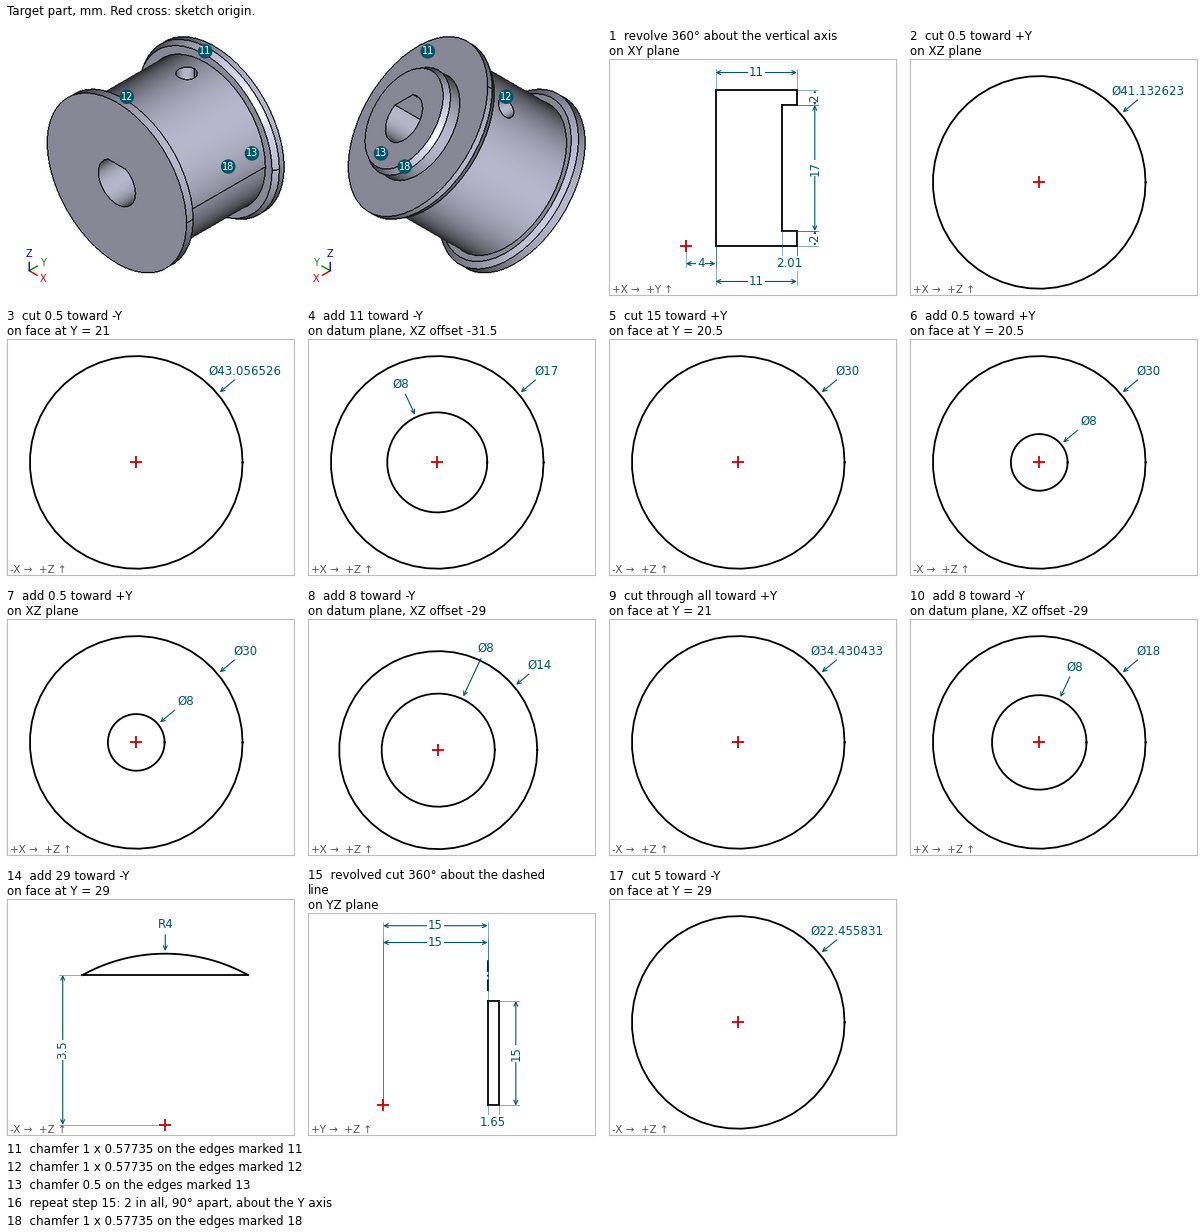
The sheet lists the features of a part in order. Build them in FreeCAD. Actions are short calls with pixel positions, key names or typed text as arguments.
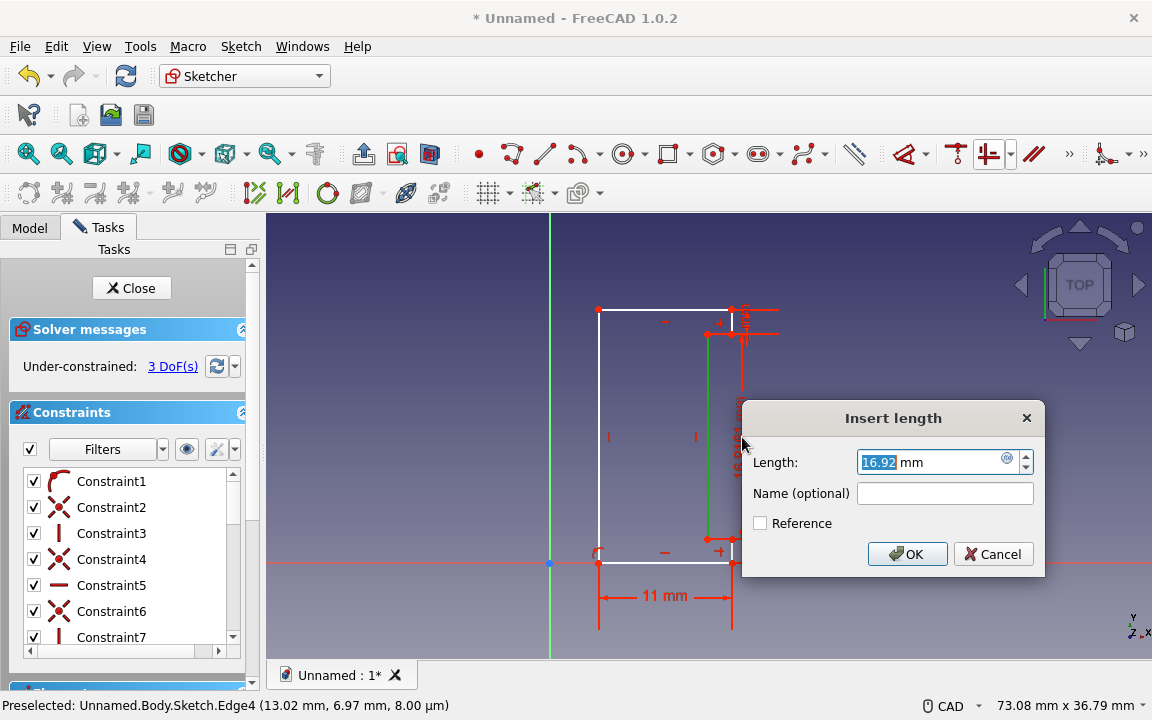
text(17)
key(Return)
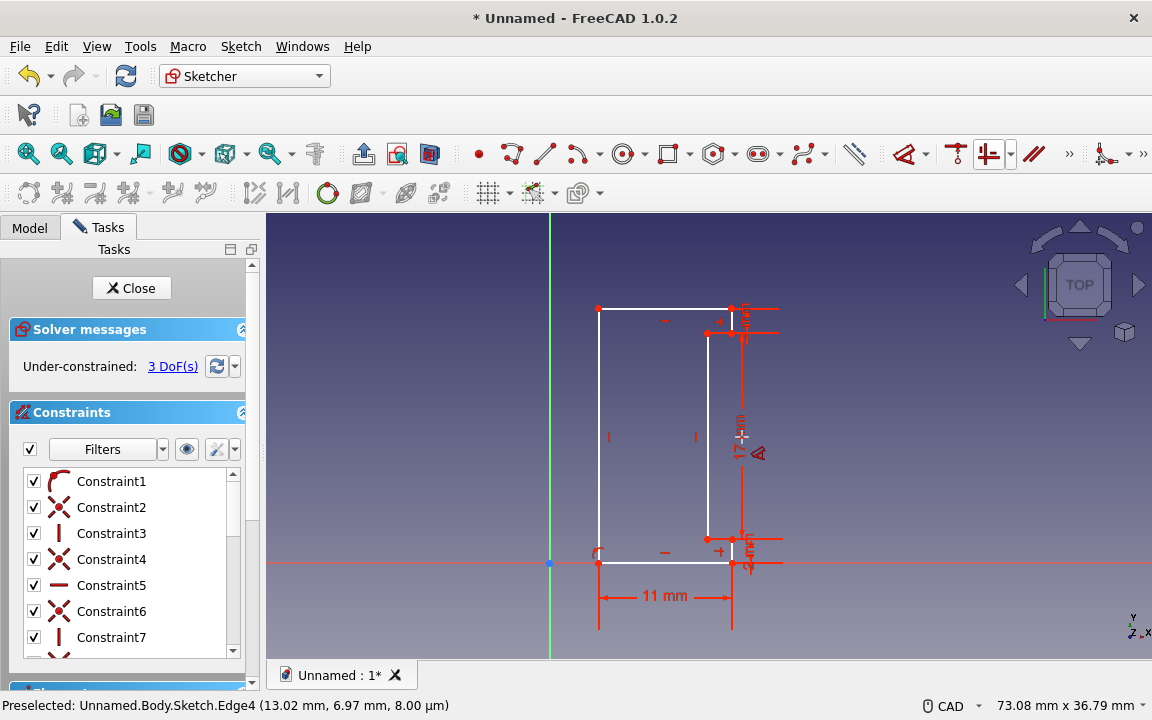
click(692, 309)
click(665, 275)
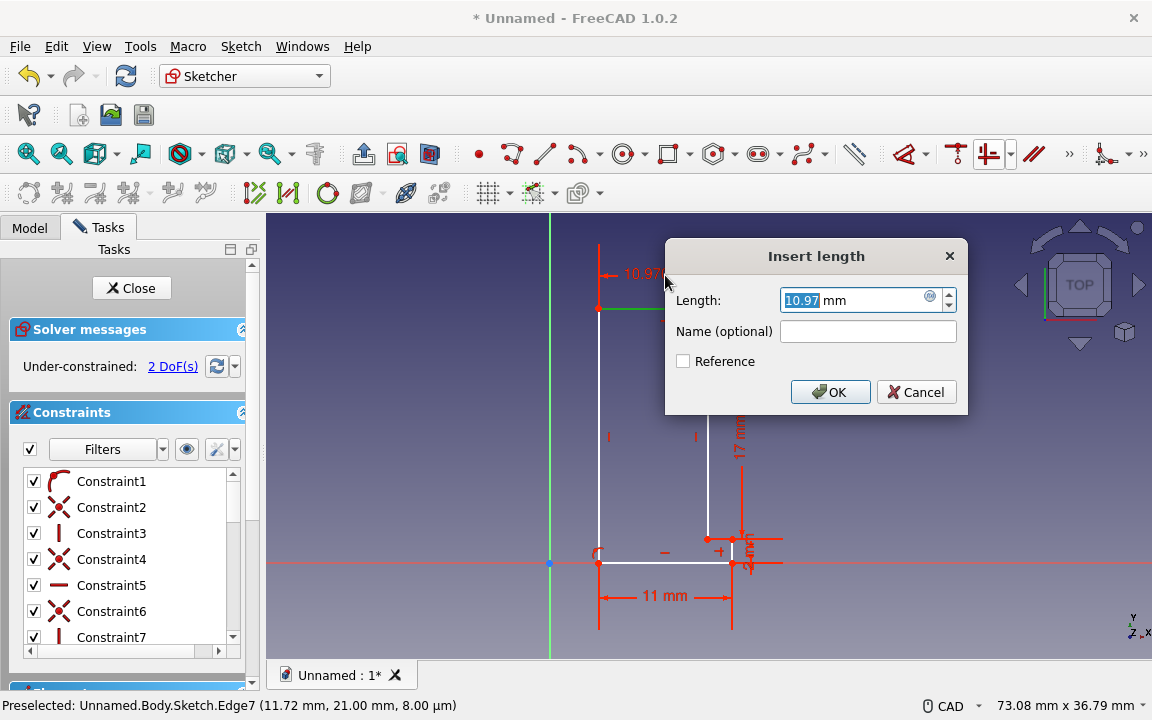
text(11)
key(Return)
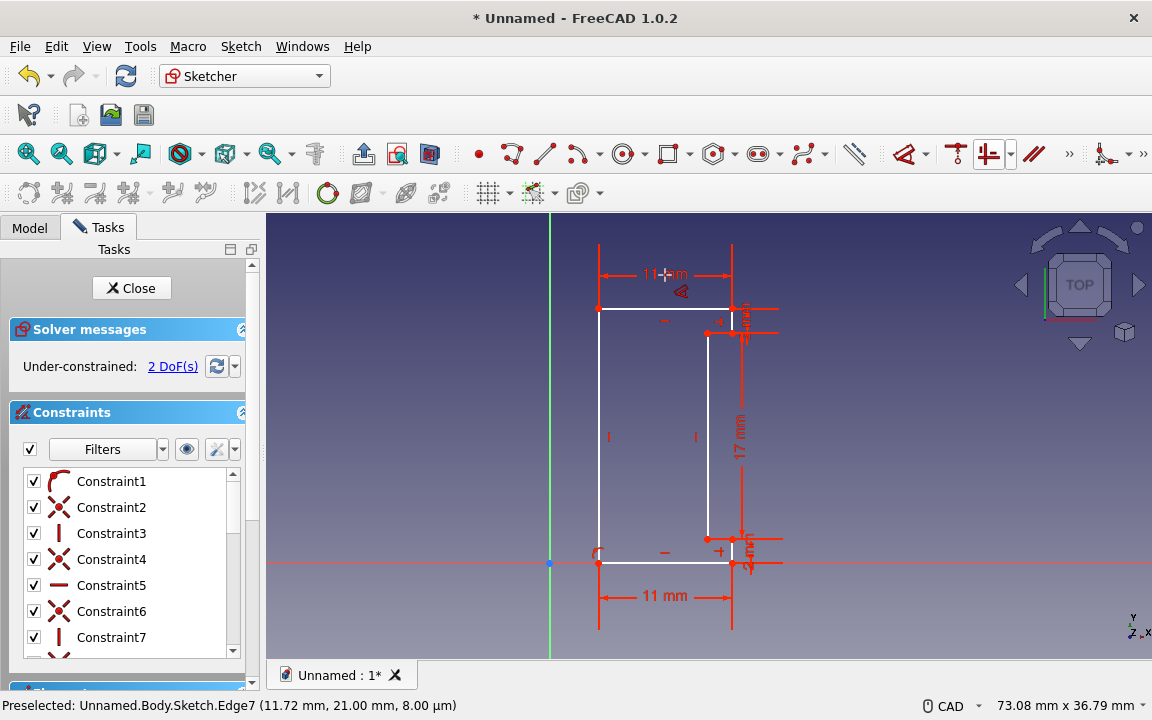
click(599, 563)
click(574, 597)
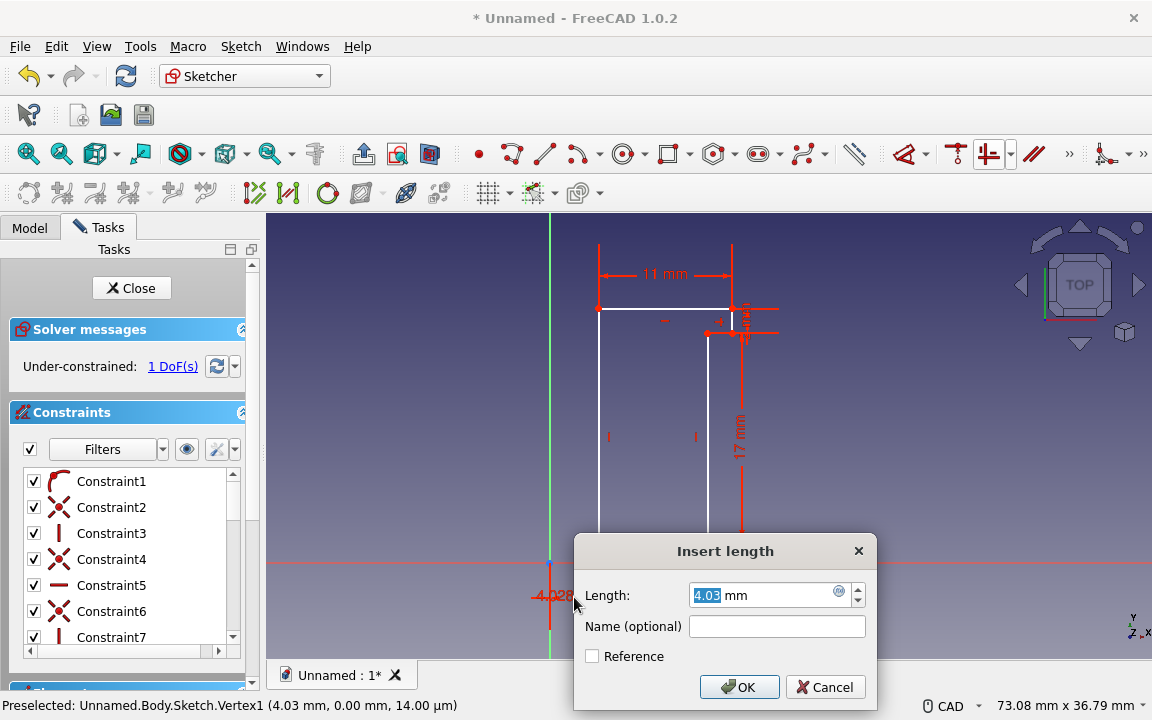
text(4)
key(Return)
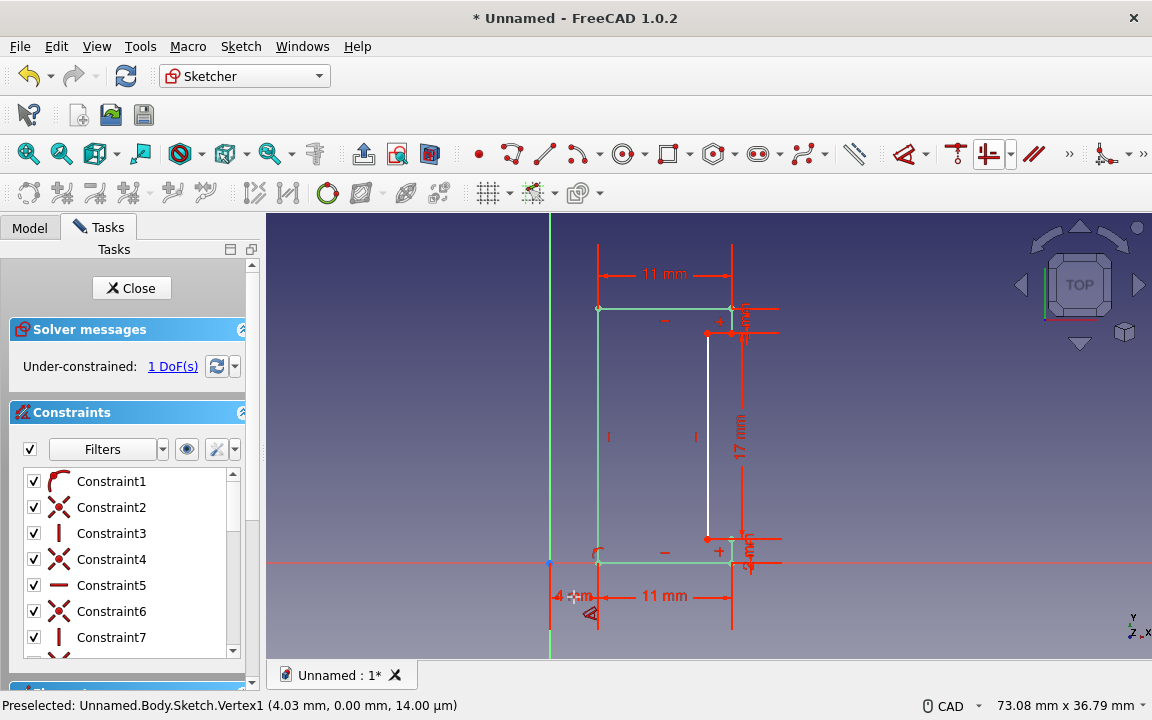
scroll(722, 539, up, 3)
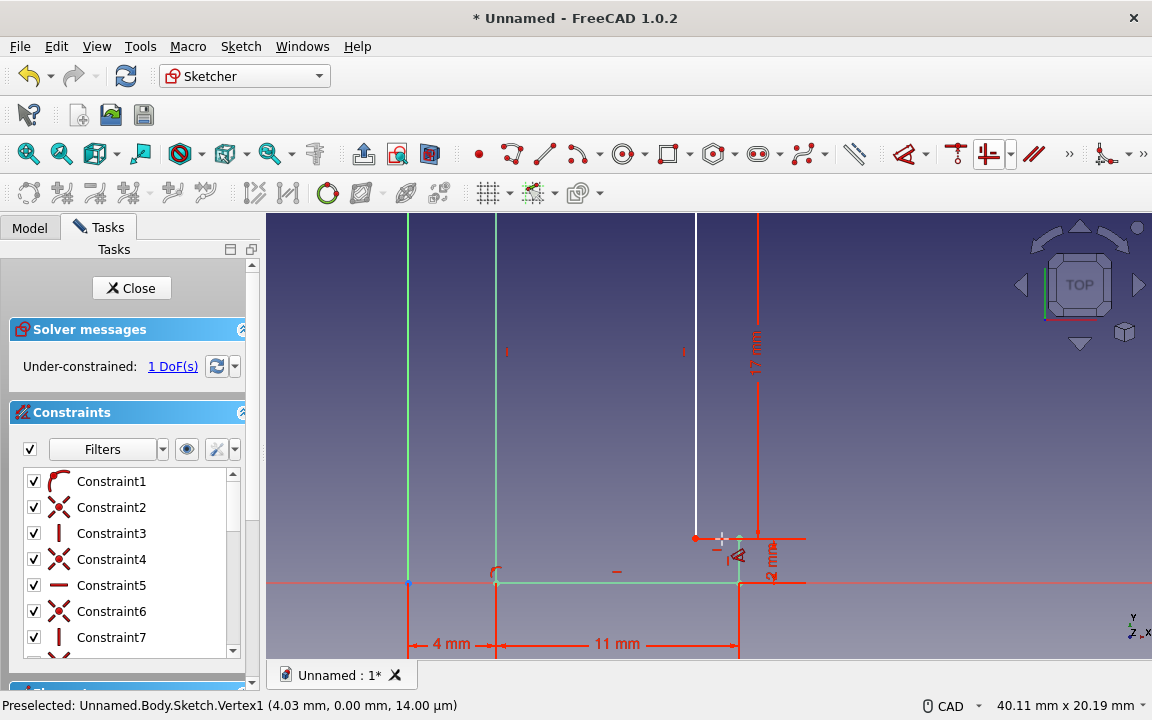
click(722, 539)
click(718, 505)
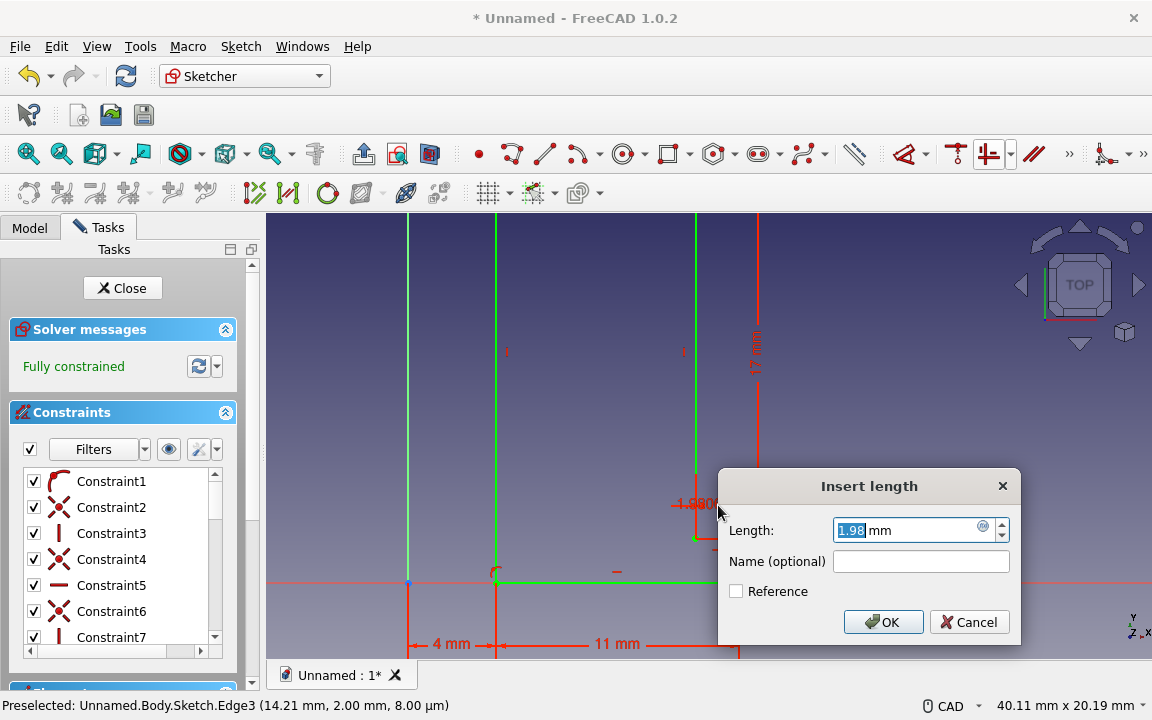
text(2.01)
key(Return)
key(Escape)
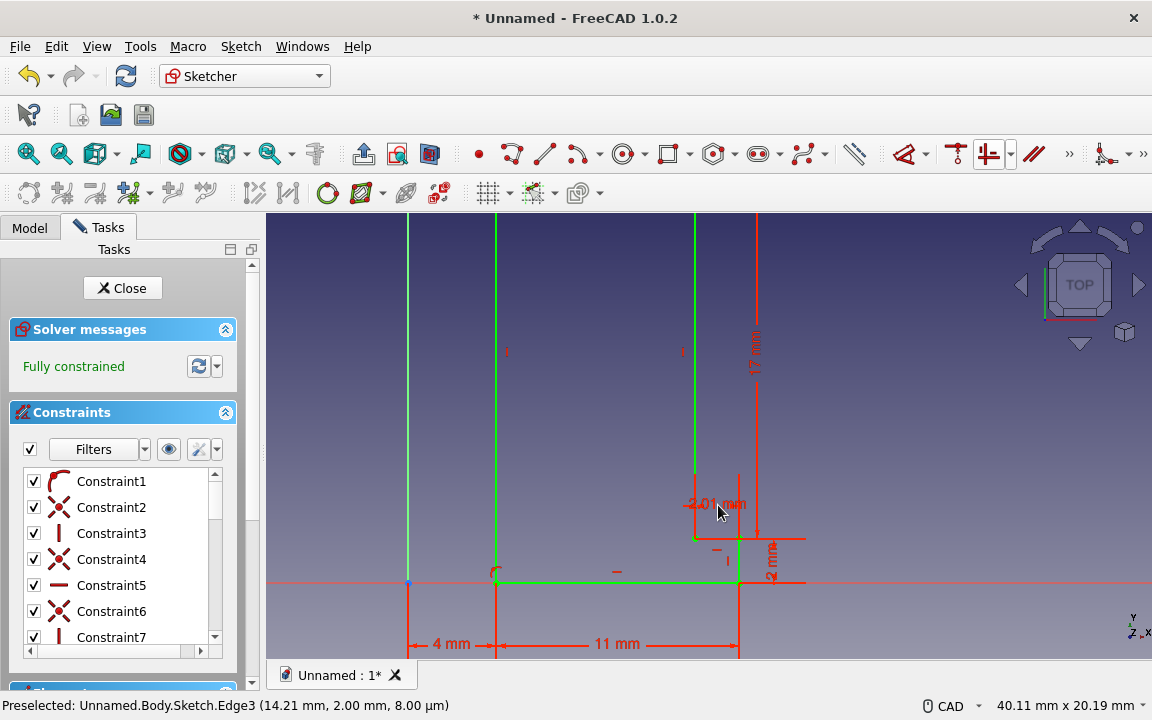
click(123, 288)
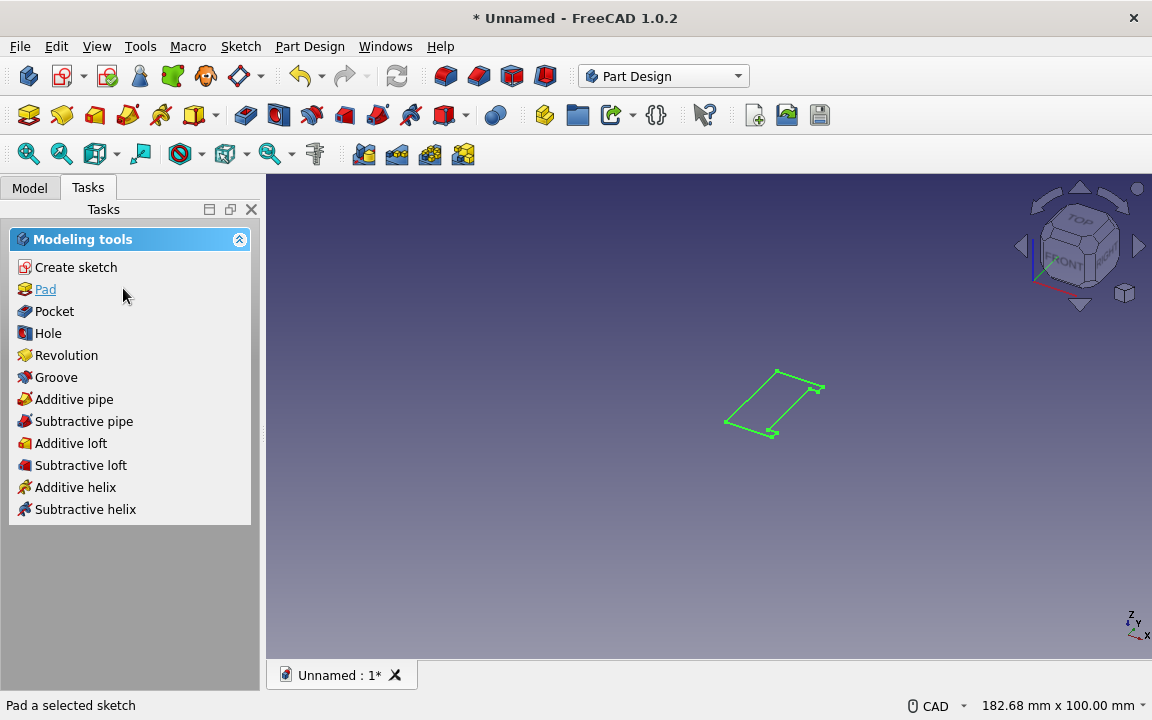
click(62, 116)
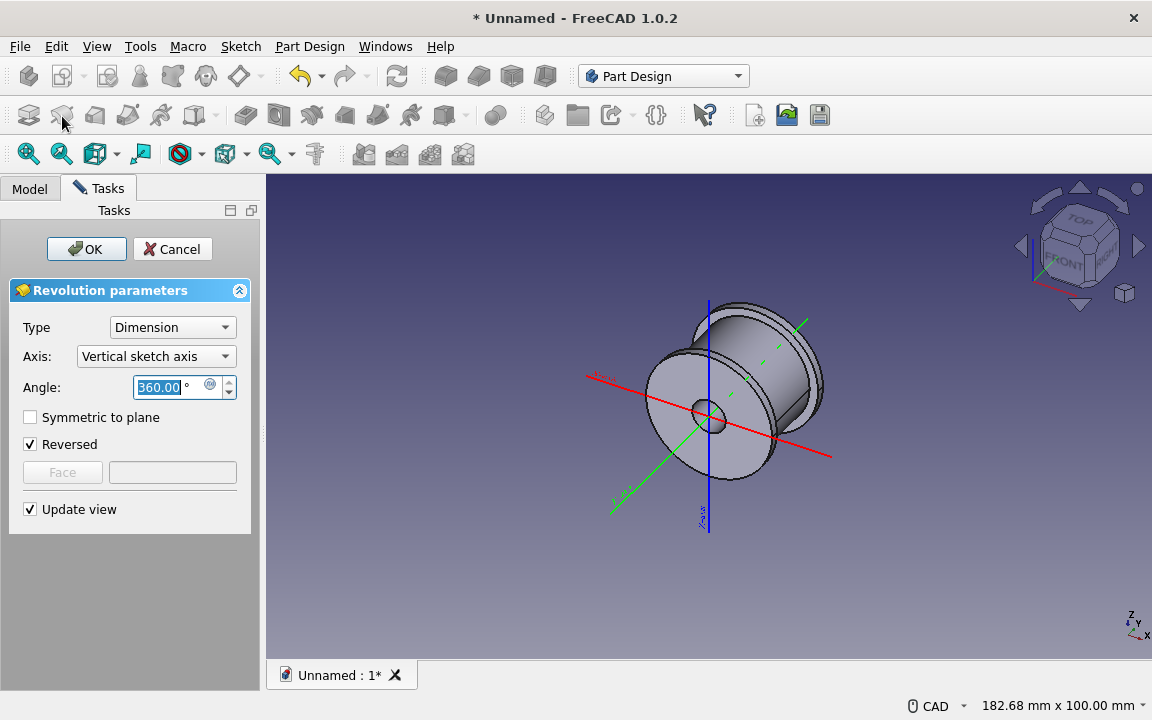
click(87, 249)